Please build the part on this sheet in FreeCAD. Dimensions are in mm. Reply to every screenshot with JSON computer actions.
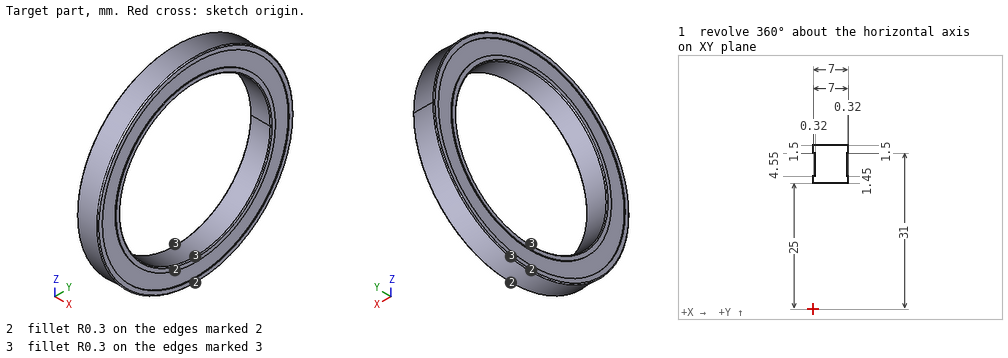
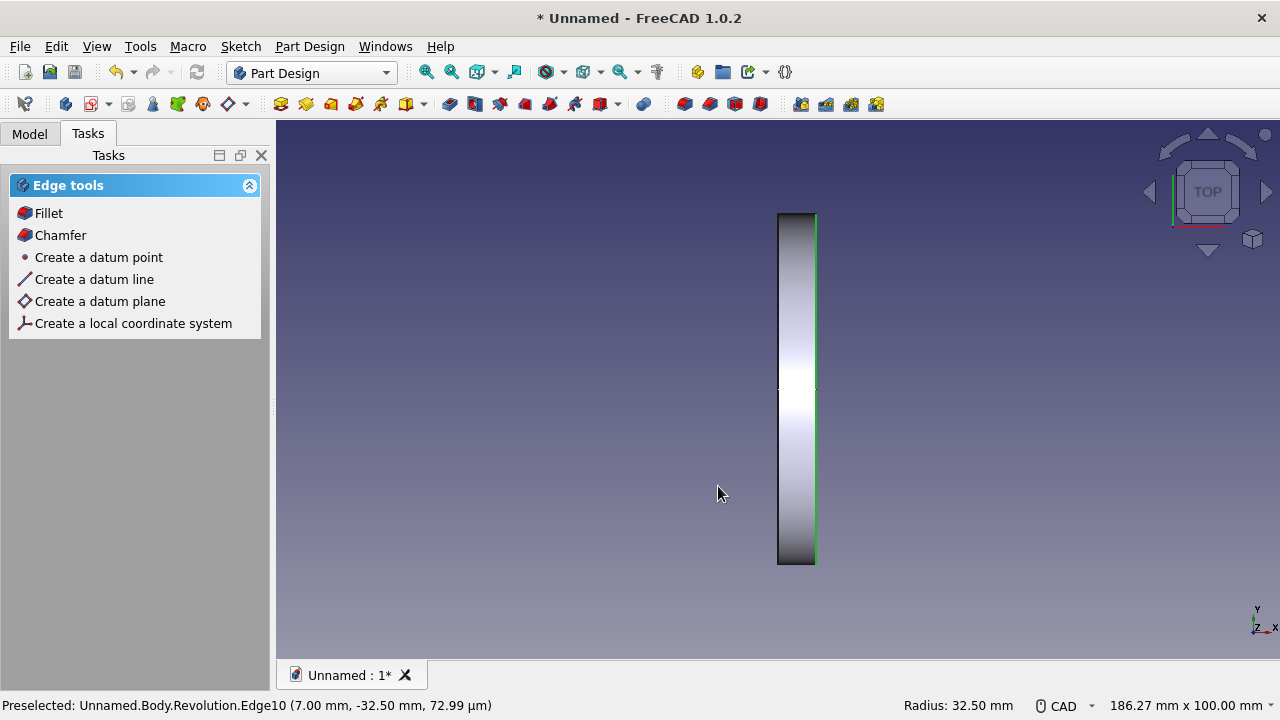
{"action": "left_click", "coordinate": [778, 530], "text": "ctrl"}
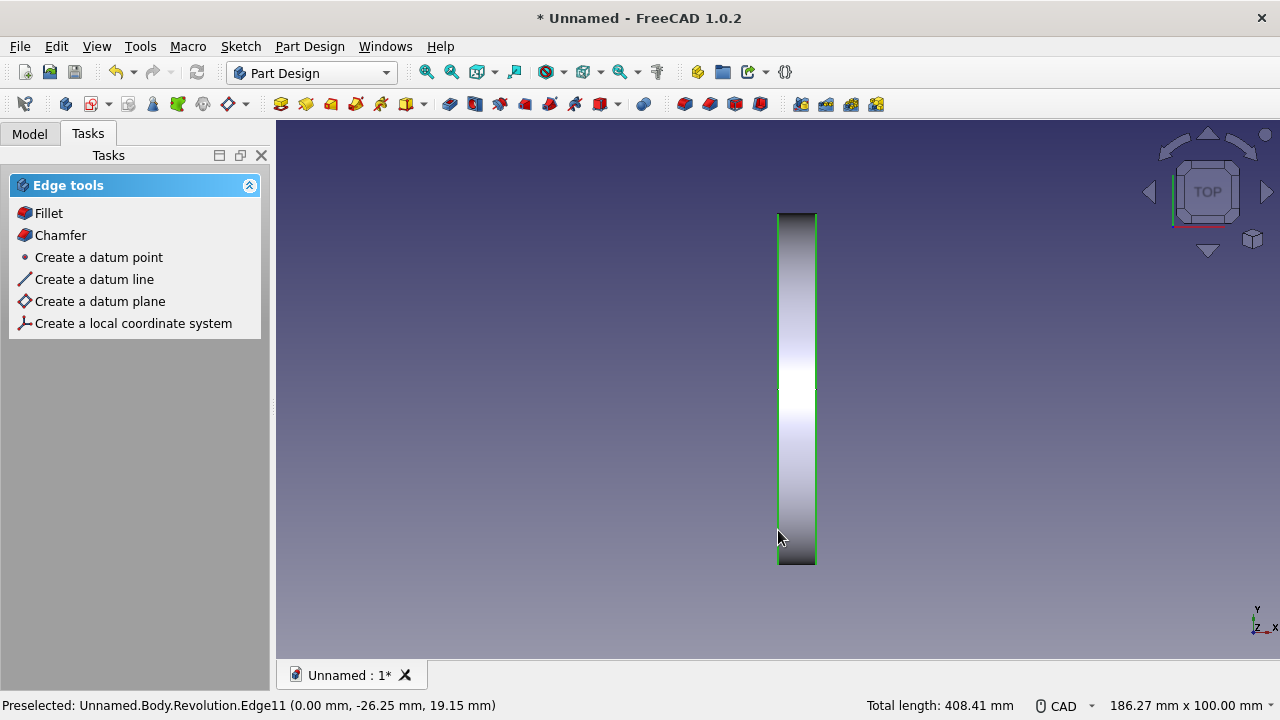
{"action": "left_click", "coordinate": [685, 104]}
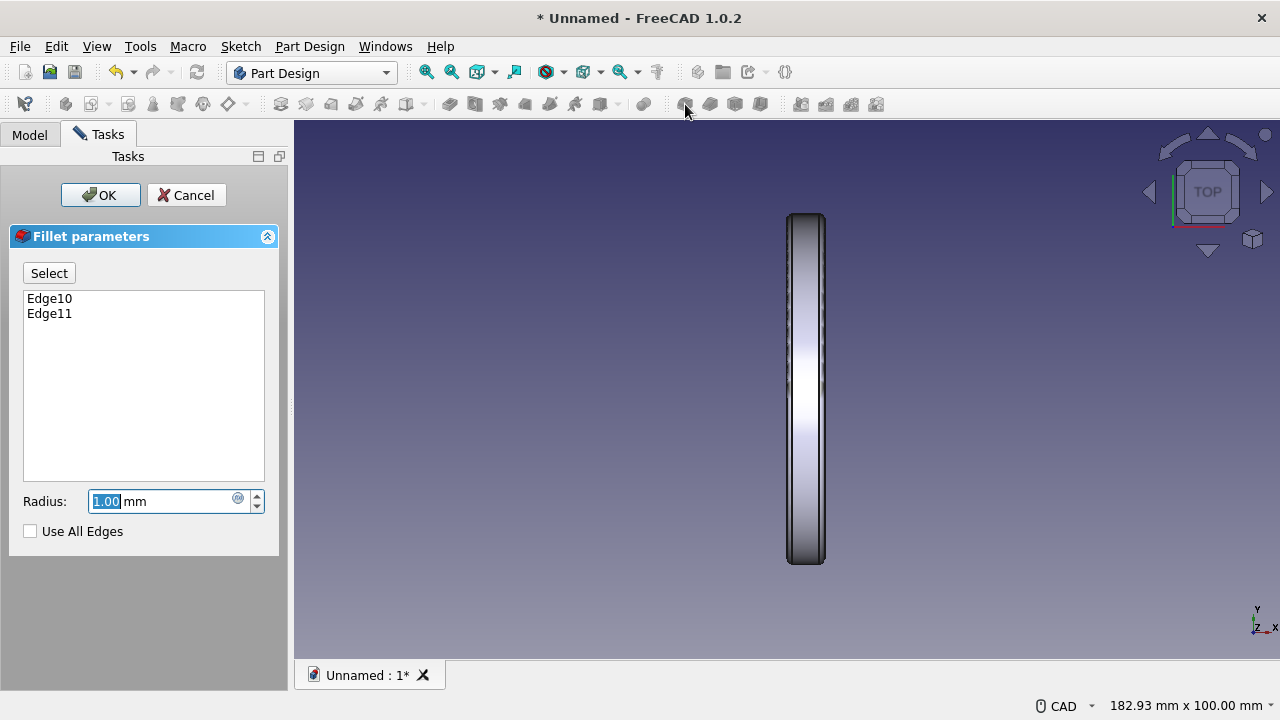
{"action": "type", "text": "0.3"}
{"action": "key", "text": "Tab"}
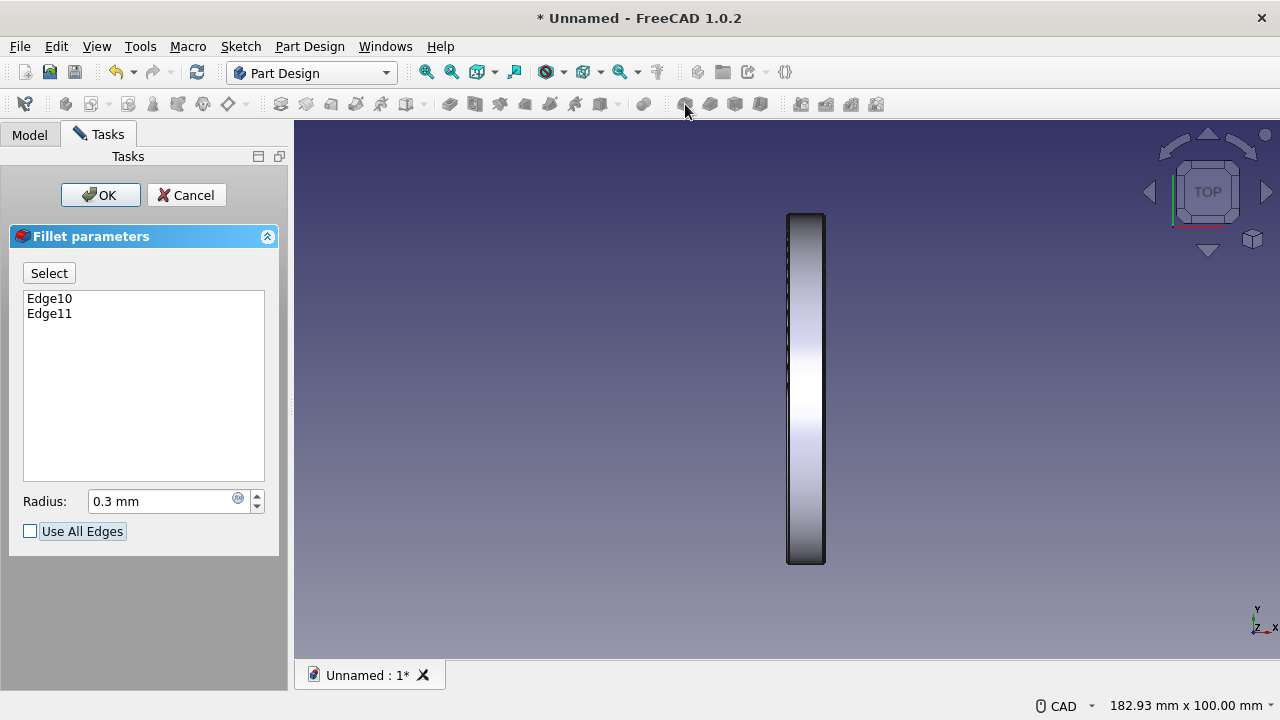
{"action": "left_click", "coordinate": [101, 195]}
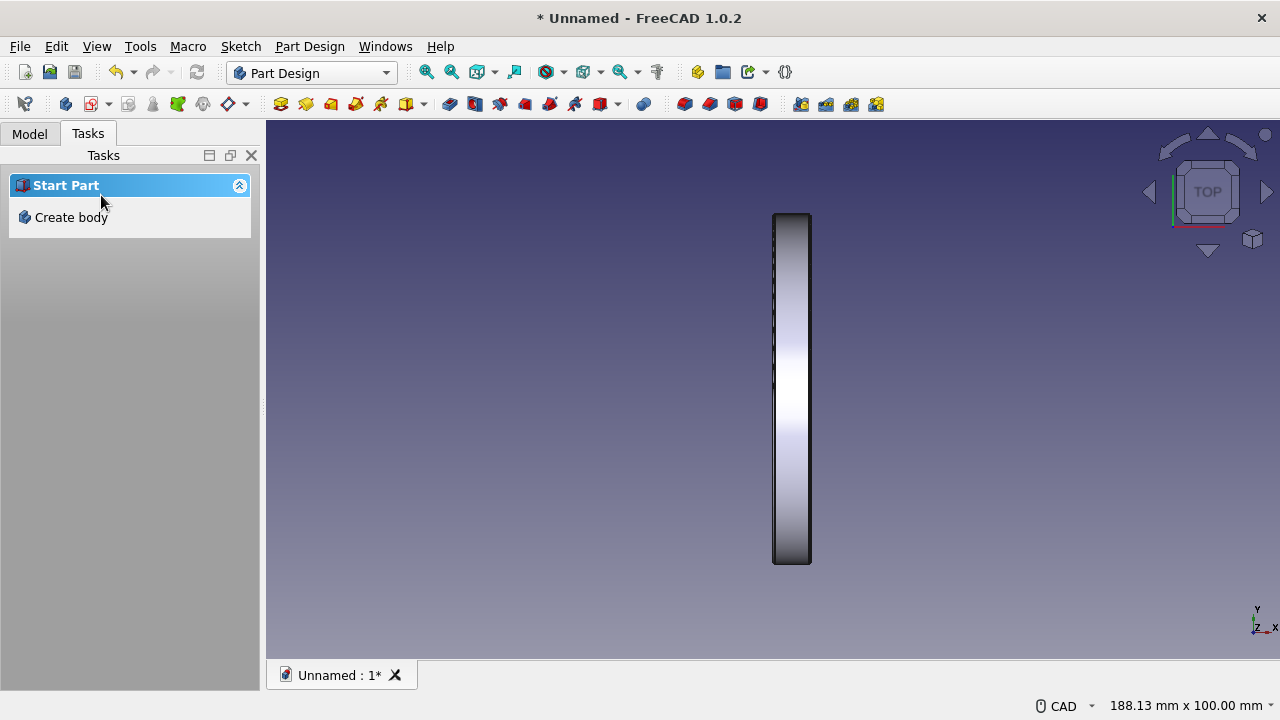
{"action": "key", "text": "0"}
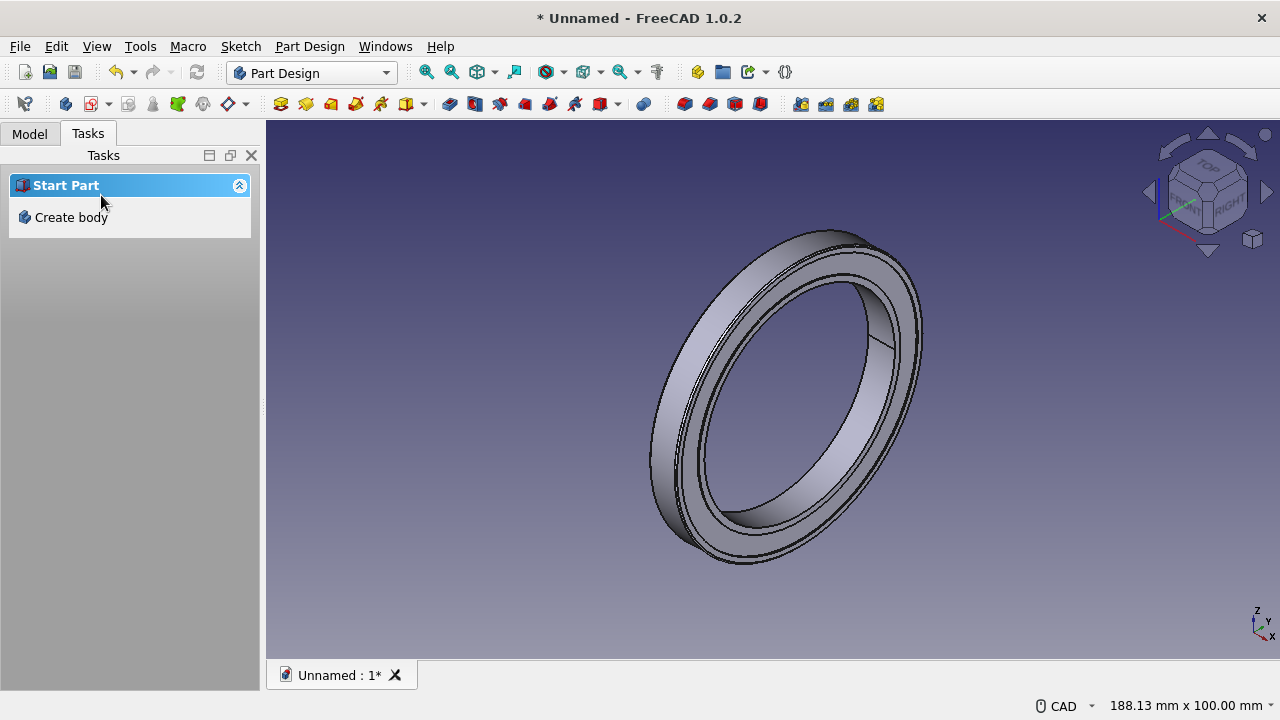
{"action": "left_click", "coordinate": [723, 513]}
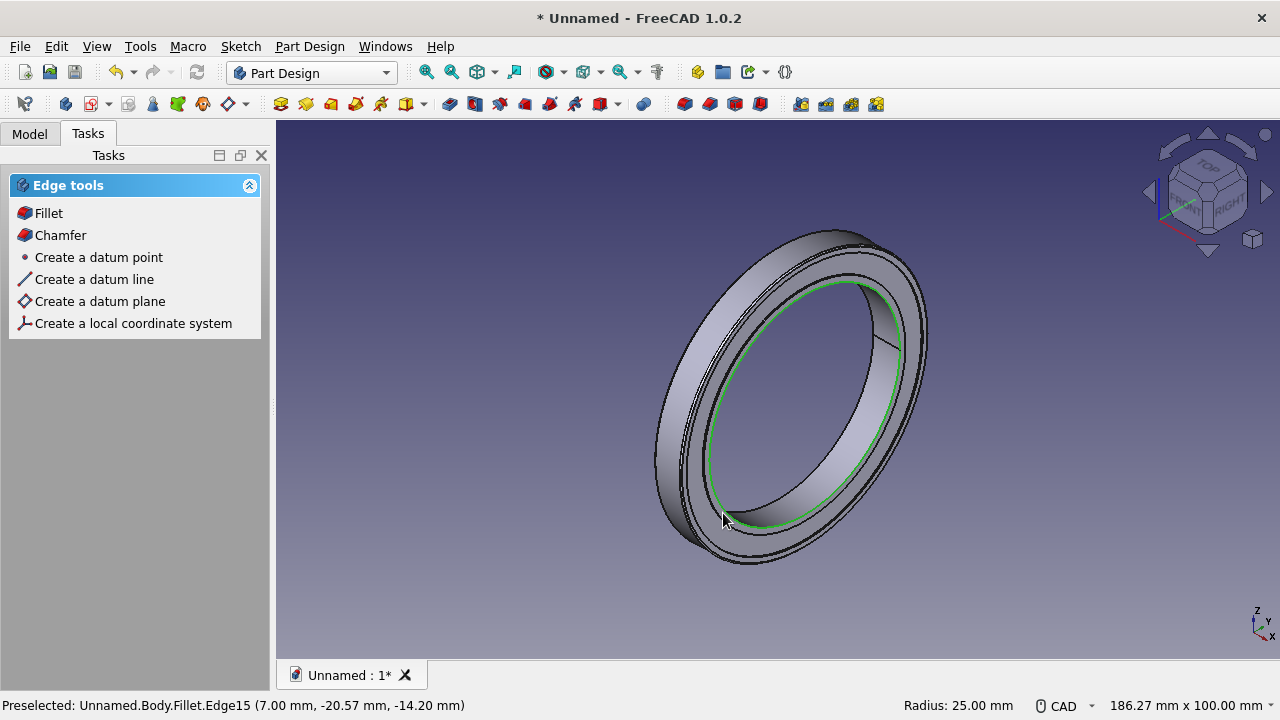
{"action": "key", "text": "2"}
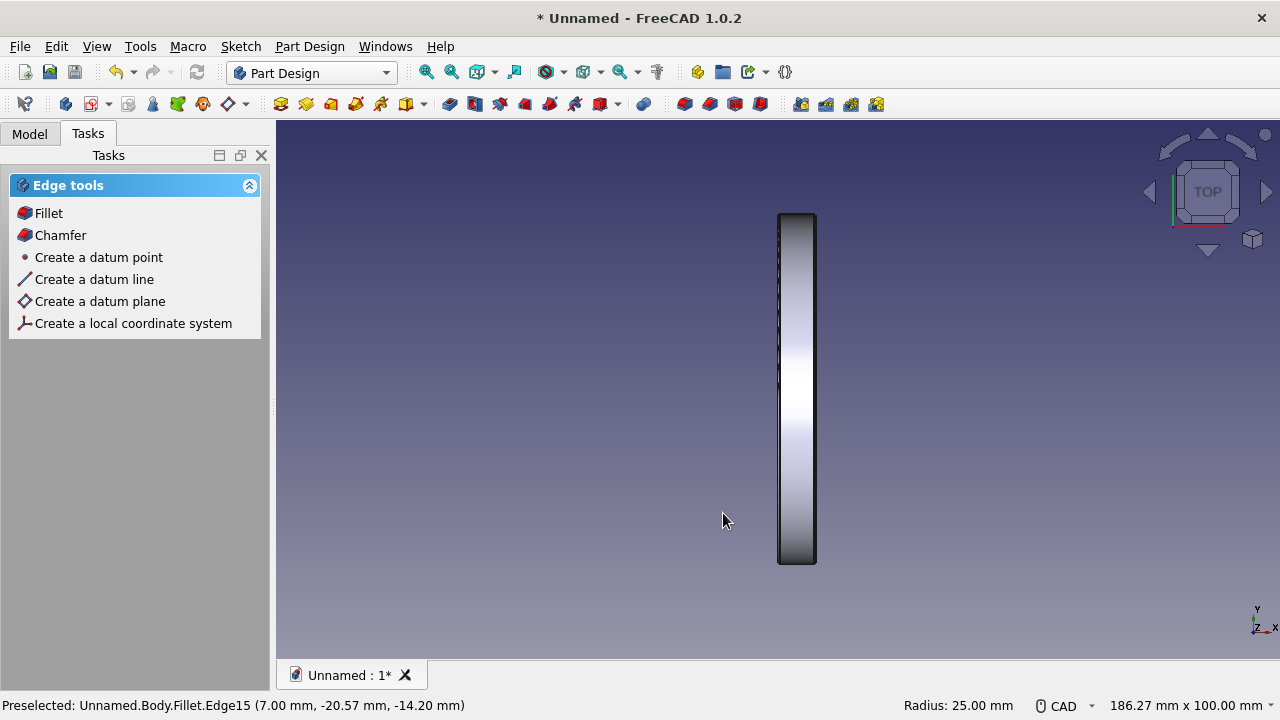
{"action": "key", "text": "1"}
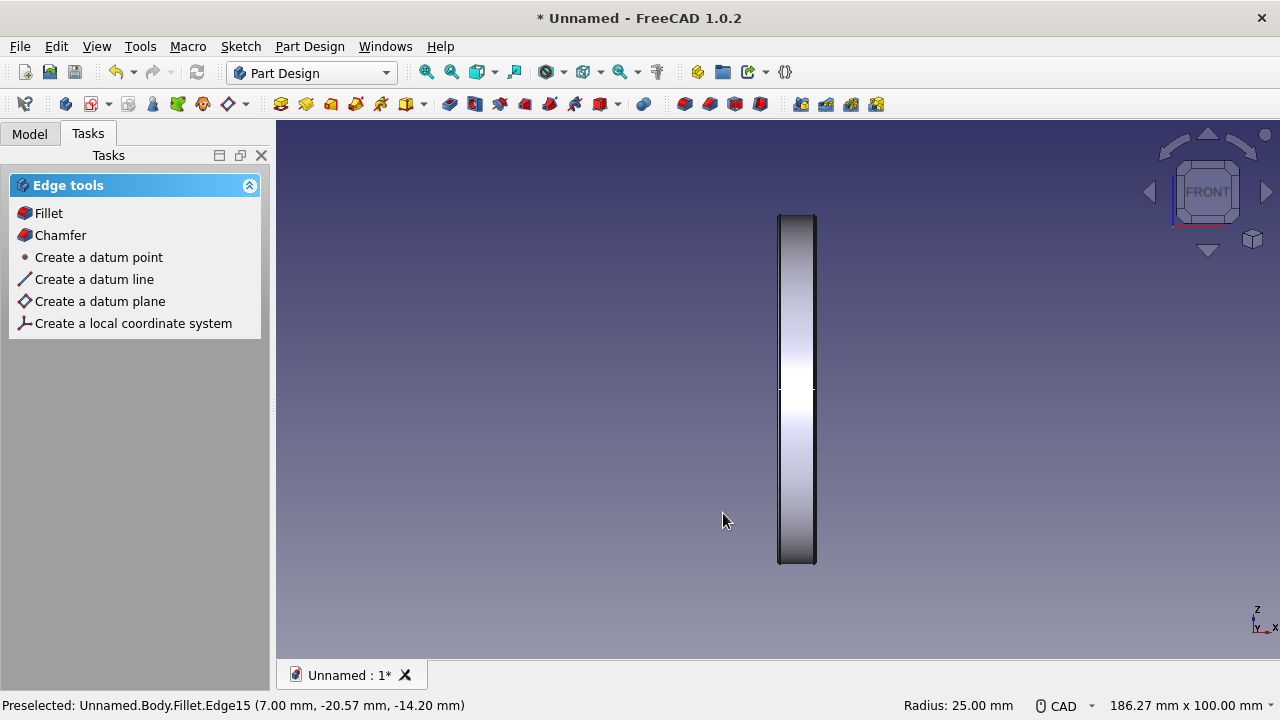
{"action": "key", "text": "3"}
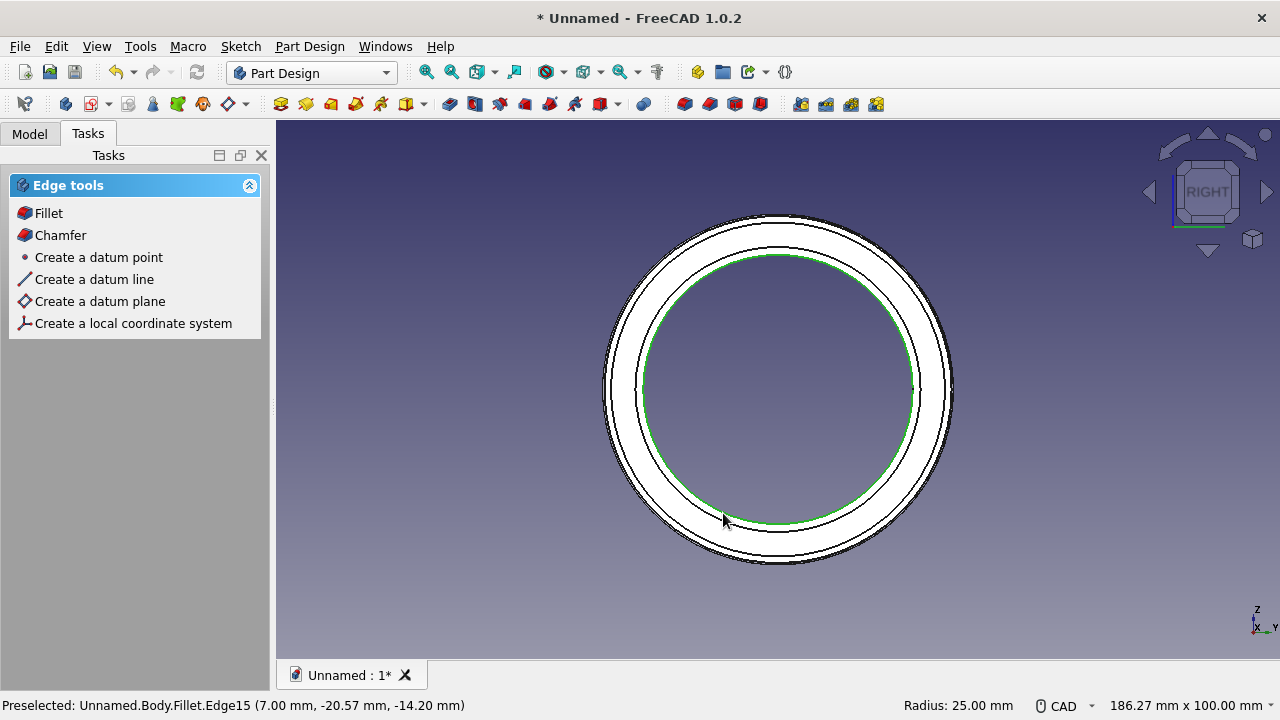
{"action": "key", "text": "5"}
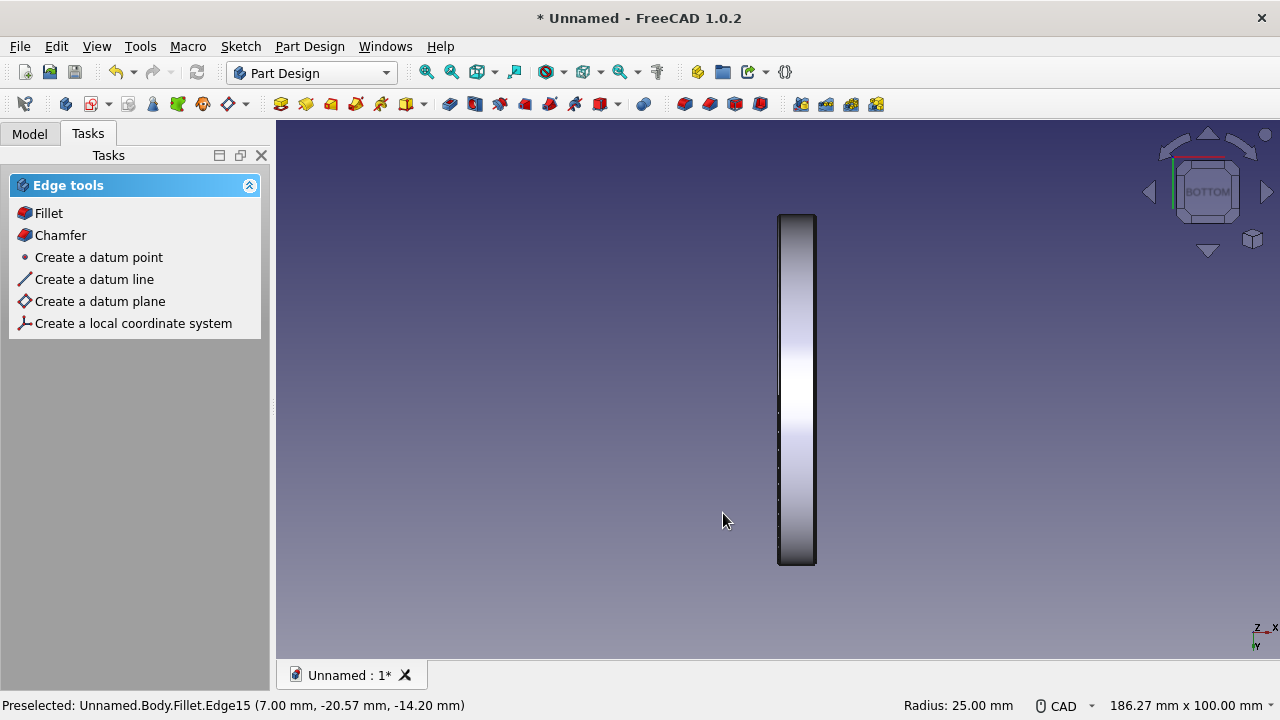
{"action": "key", "text": "4"}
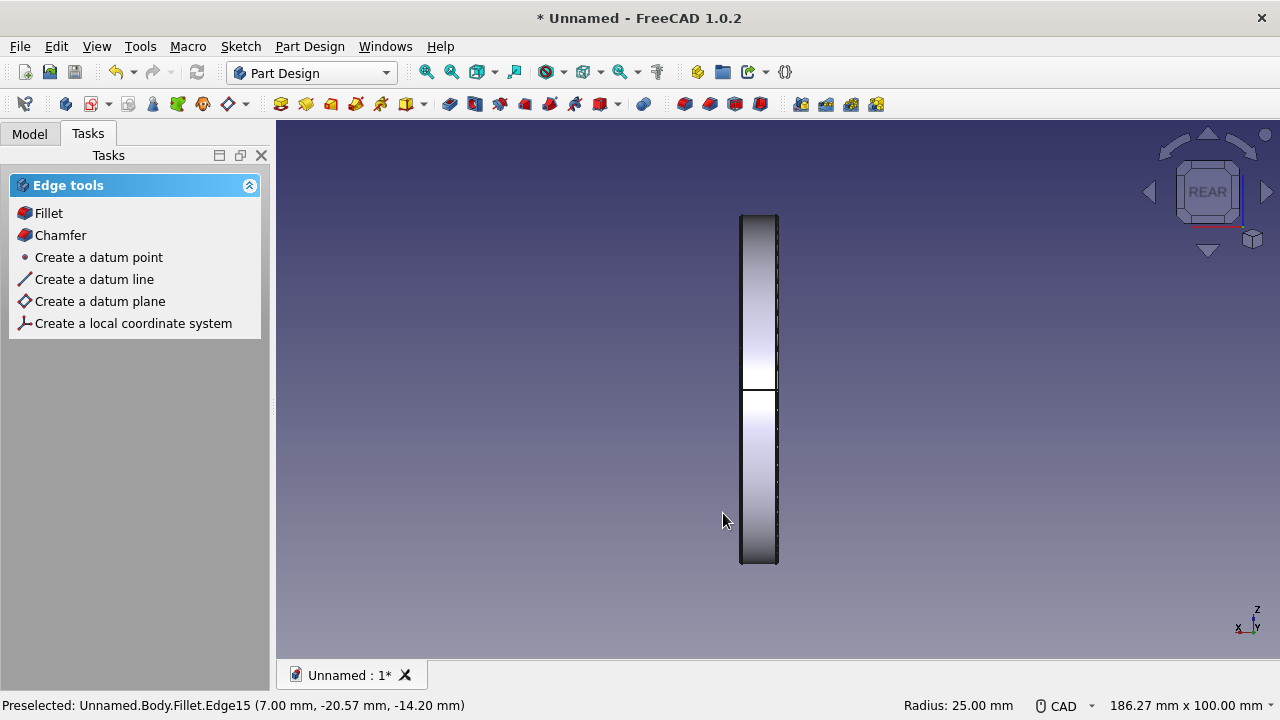
{"action": "key", "text": "6"}